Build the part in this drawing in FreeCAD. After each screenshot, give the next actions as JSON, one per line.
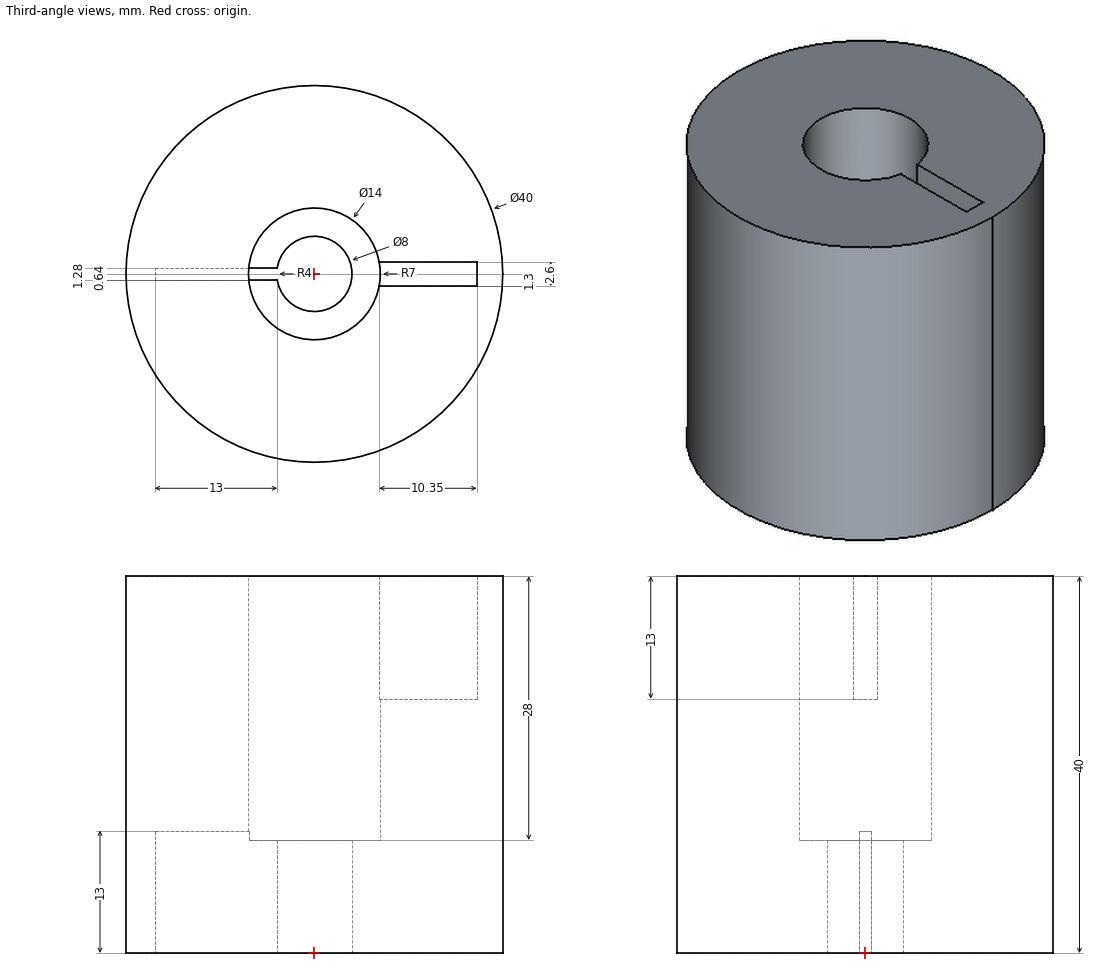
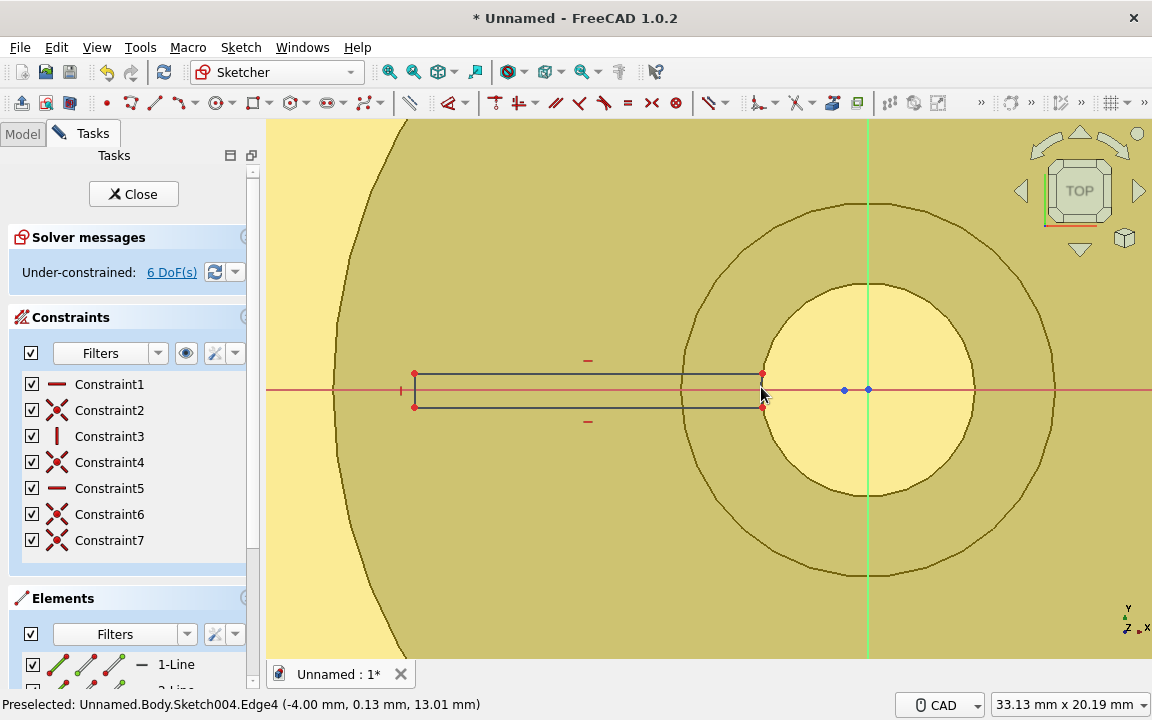
{"action": "left_click_drag", "start_coordinate": [835, 380], "coordinate": [878, 401]}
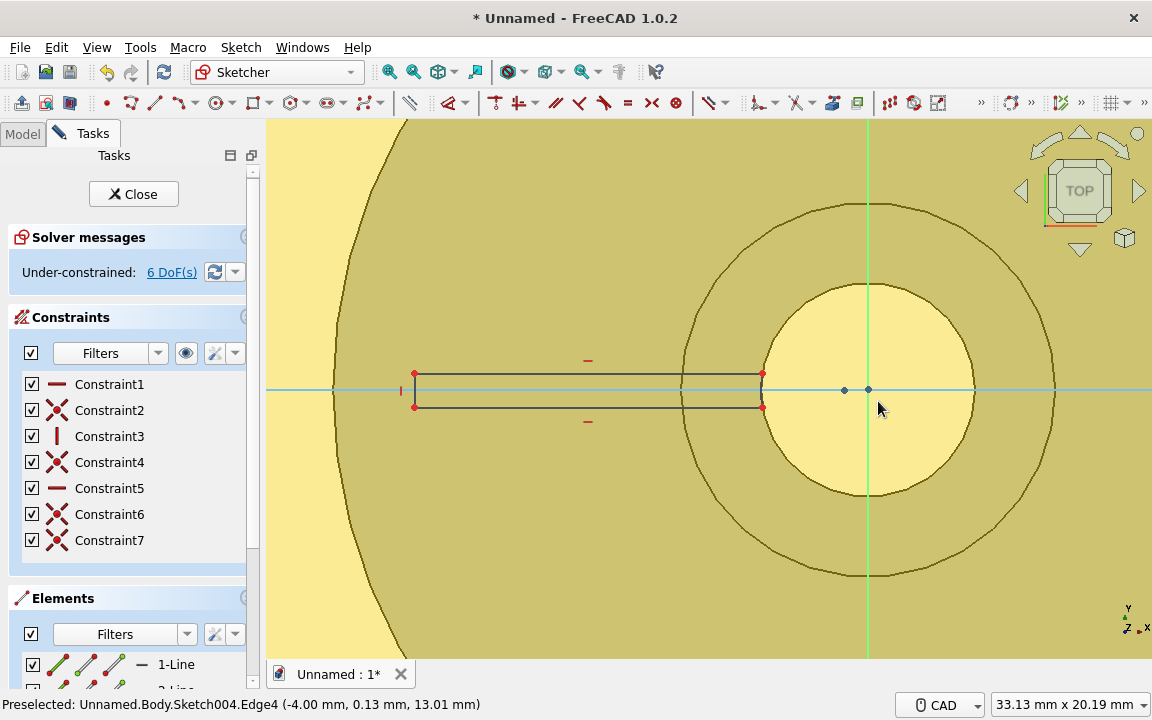
{"action": "key", "text": "c"}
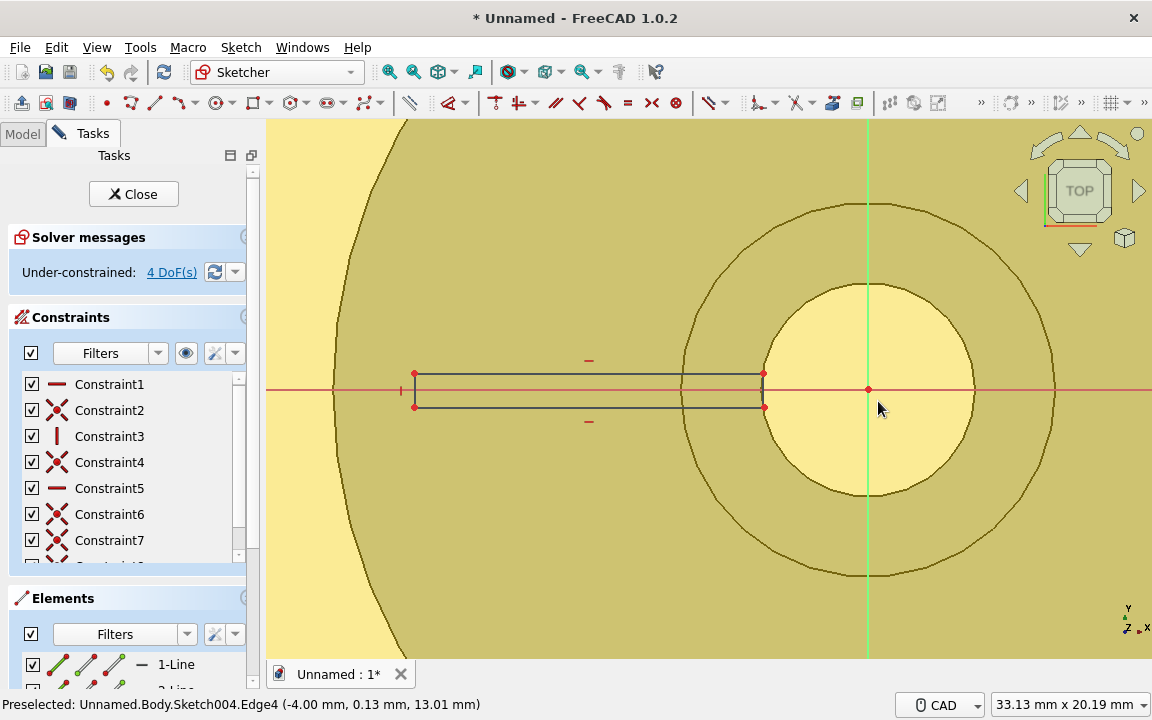
{"action": "key", "text": "d"}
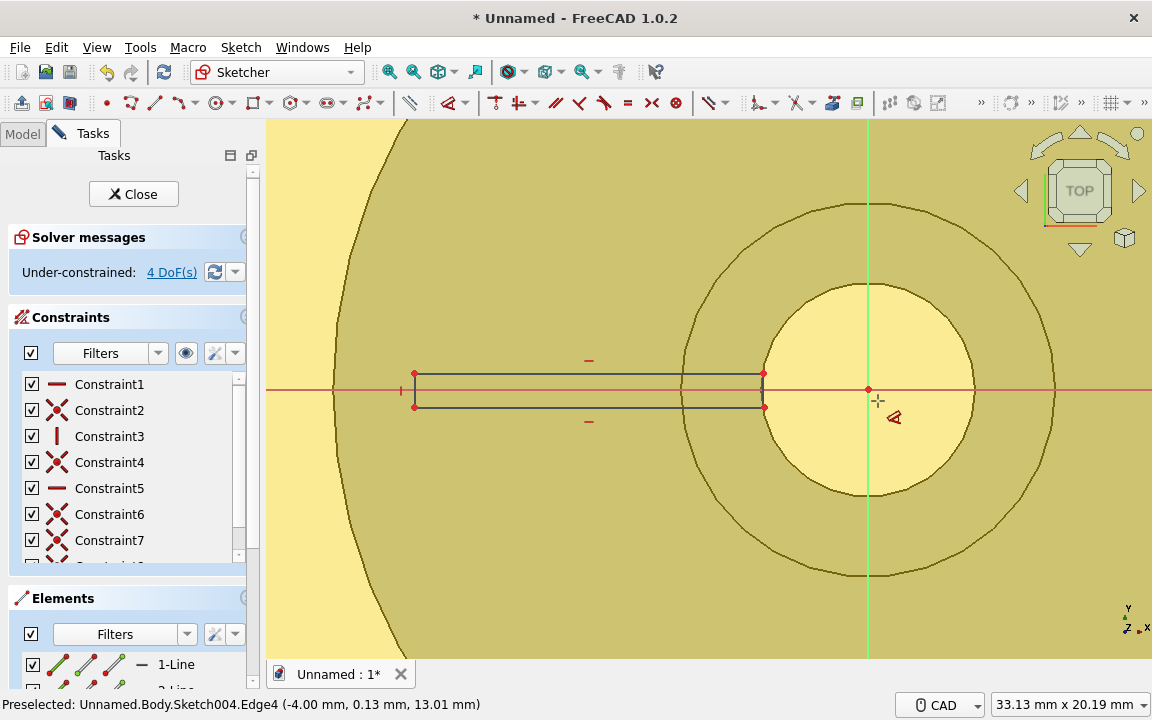
{"action": "left_click", "coordinate": [763, 391]}
{"action": "left_click", "coordinate": [747, 325]}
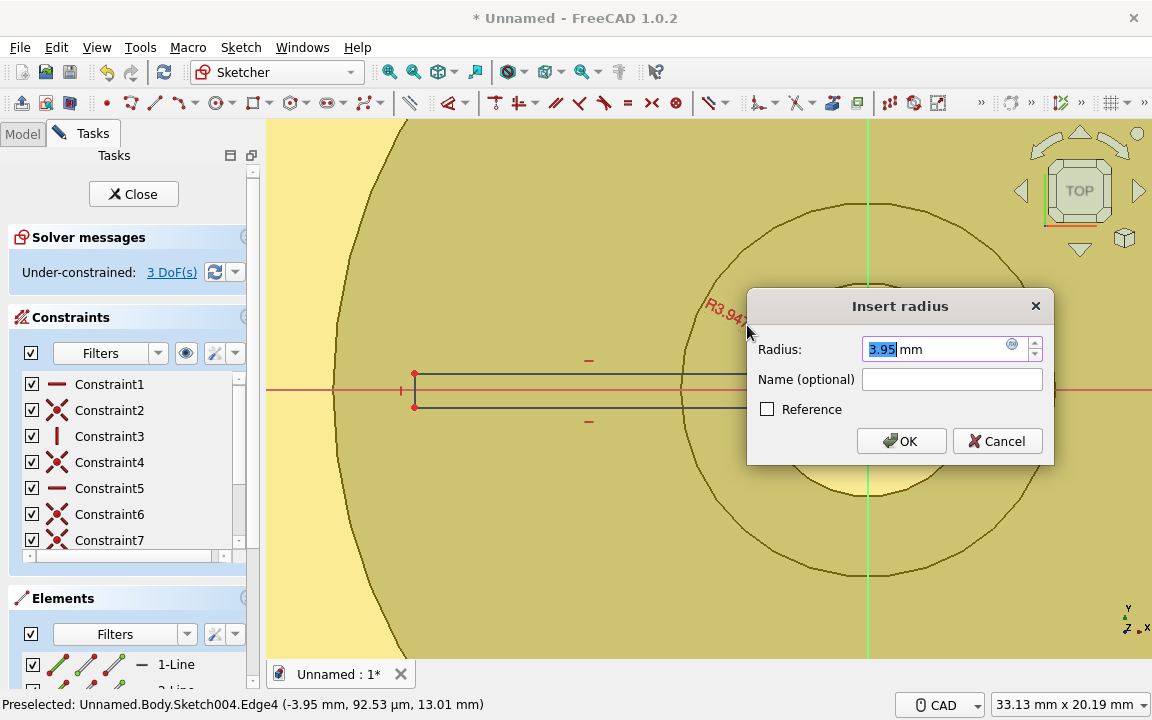
{"action": "type", "text": "4"}
{"action": "key", "text": "Return"}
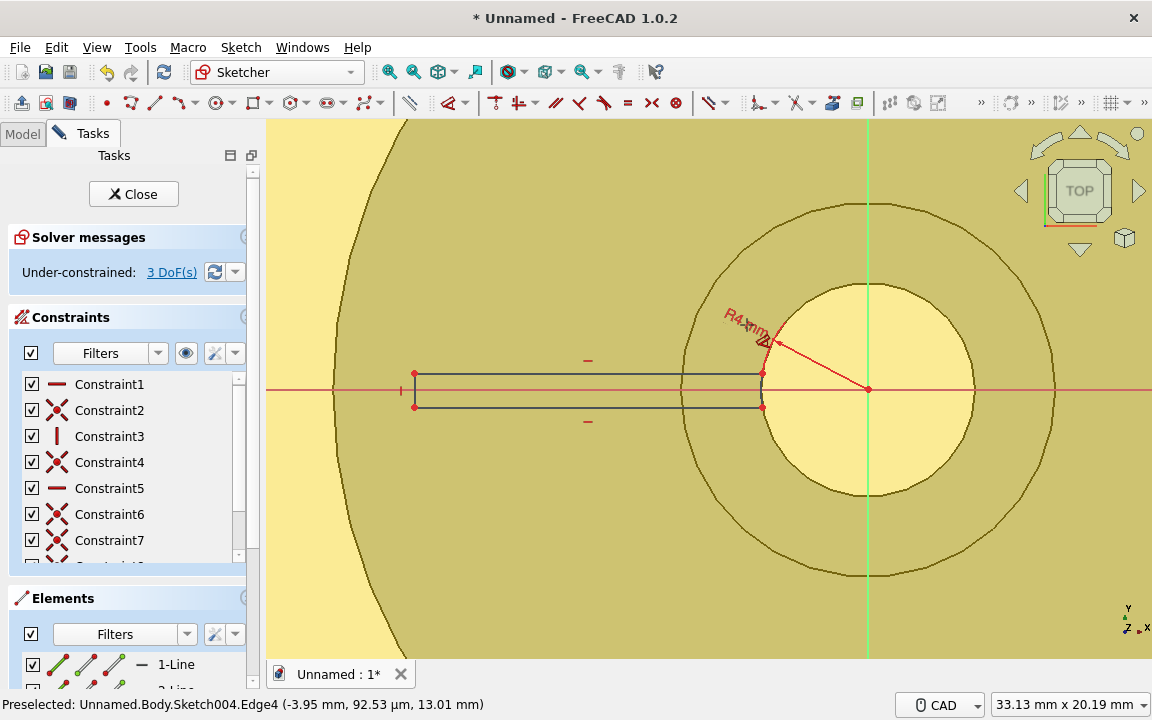
{"action": "left_click", "coordinate": [658, 408]}
{"action": "left_click", "coordinate": [589, 442]}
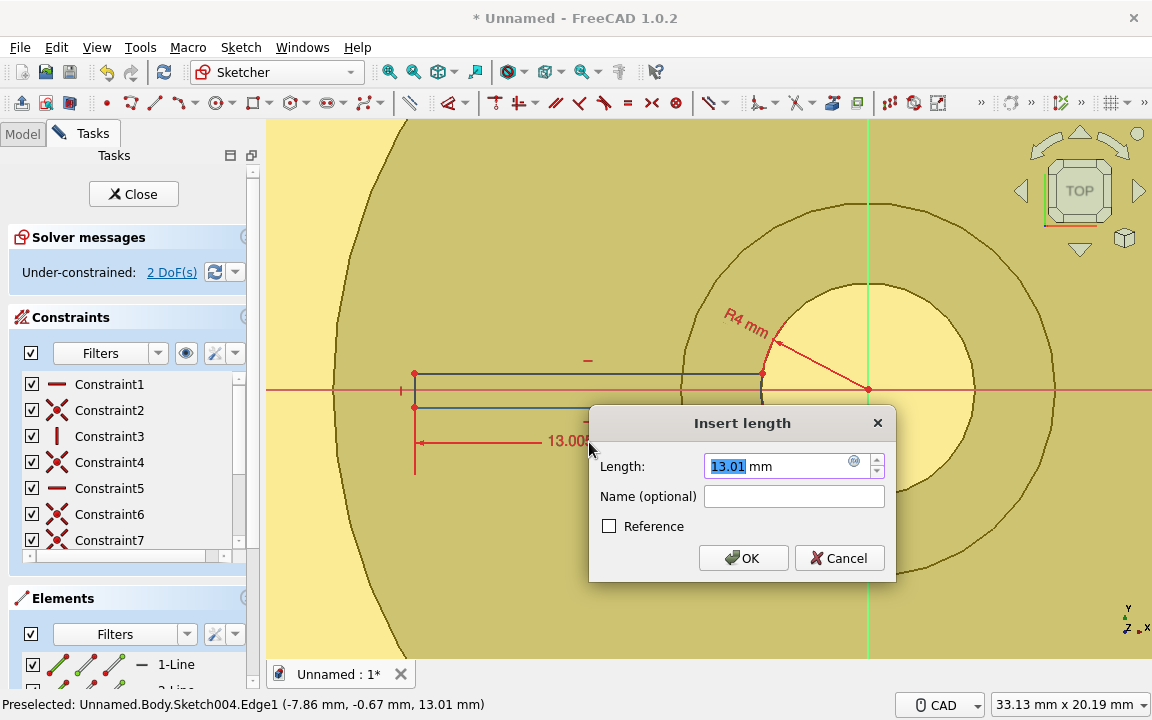
{"action": "type", "text": "13"}
{"action": "key", "text": "Return"}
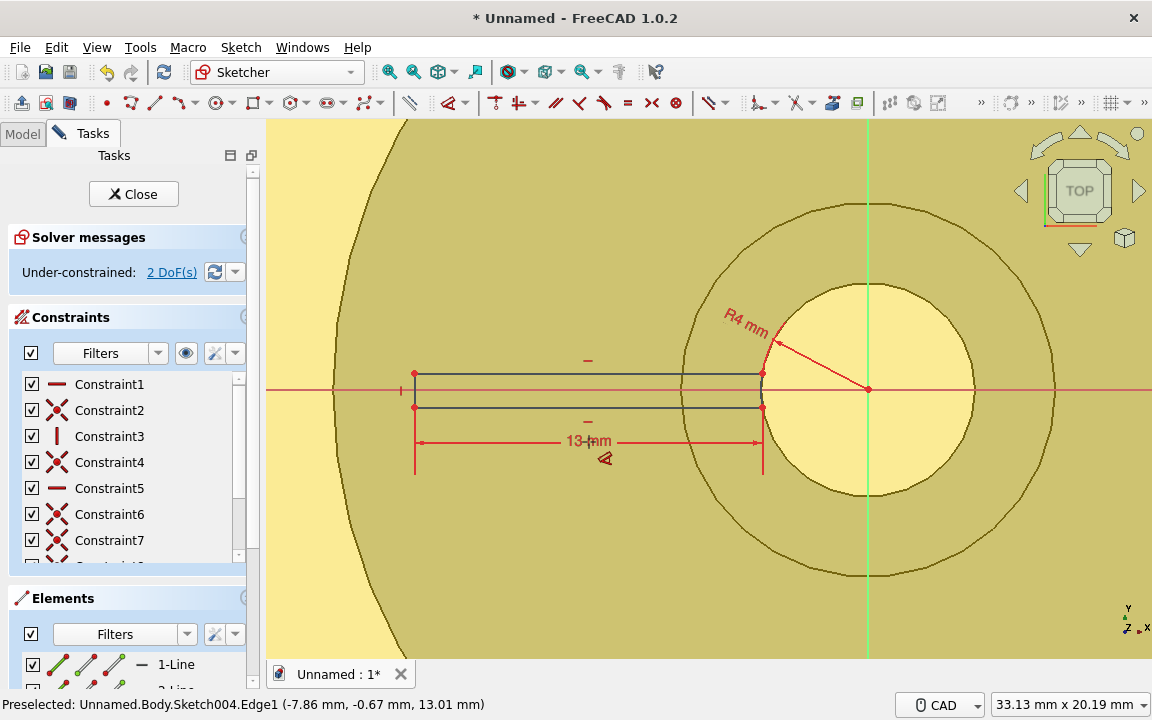
{"action": "left_click", "coordinate": [415, 387]}
{"action": "left_click", "coordinate": [381, 383]}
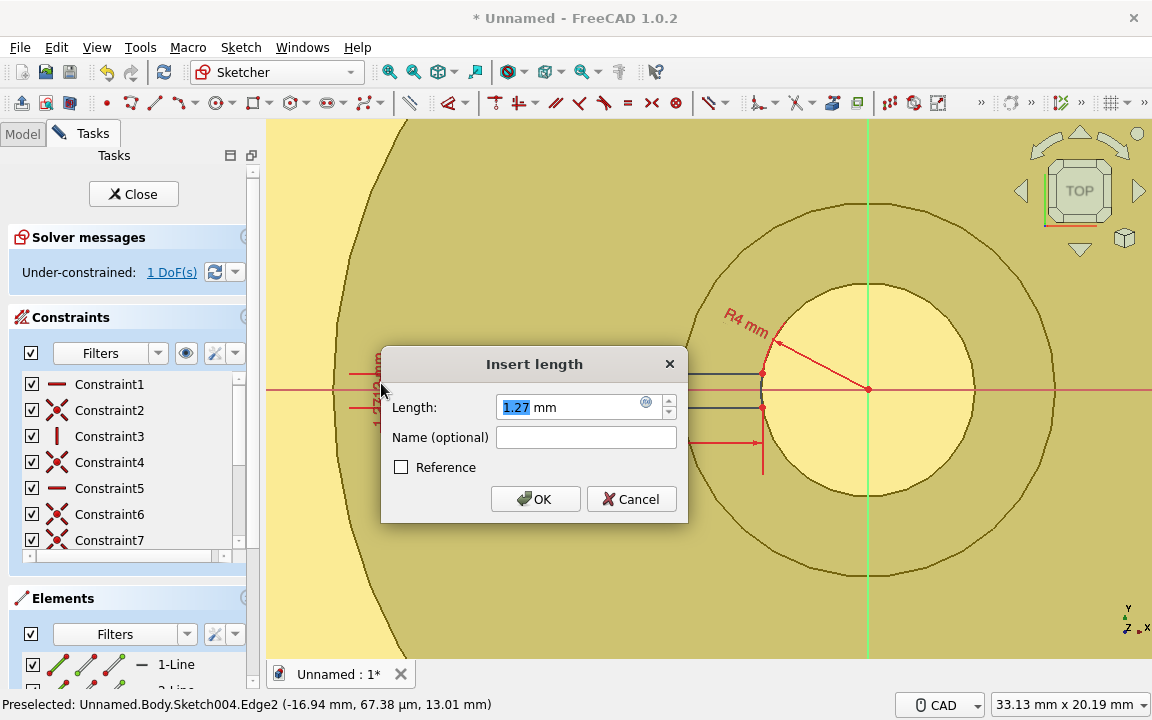
{"action": "type", "text": "1.28"}
{"action": "key", "text": "Return"}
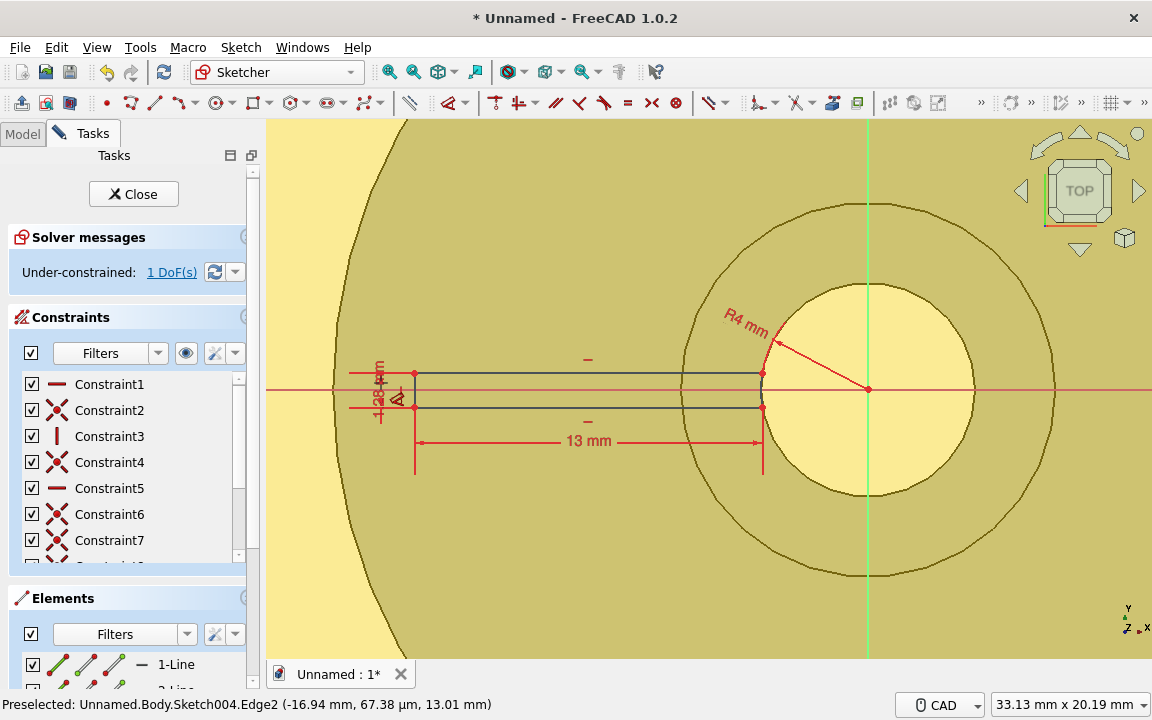
{"action": "scroll", "coordinate": [763, 408], "scroll_direction": "up", "scroll_amount": 5}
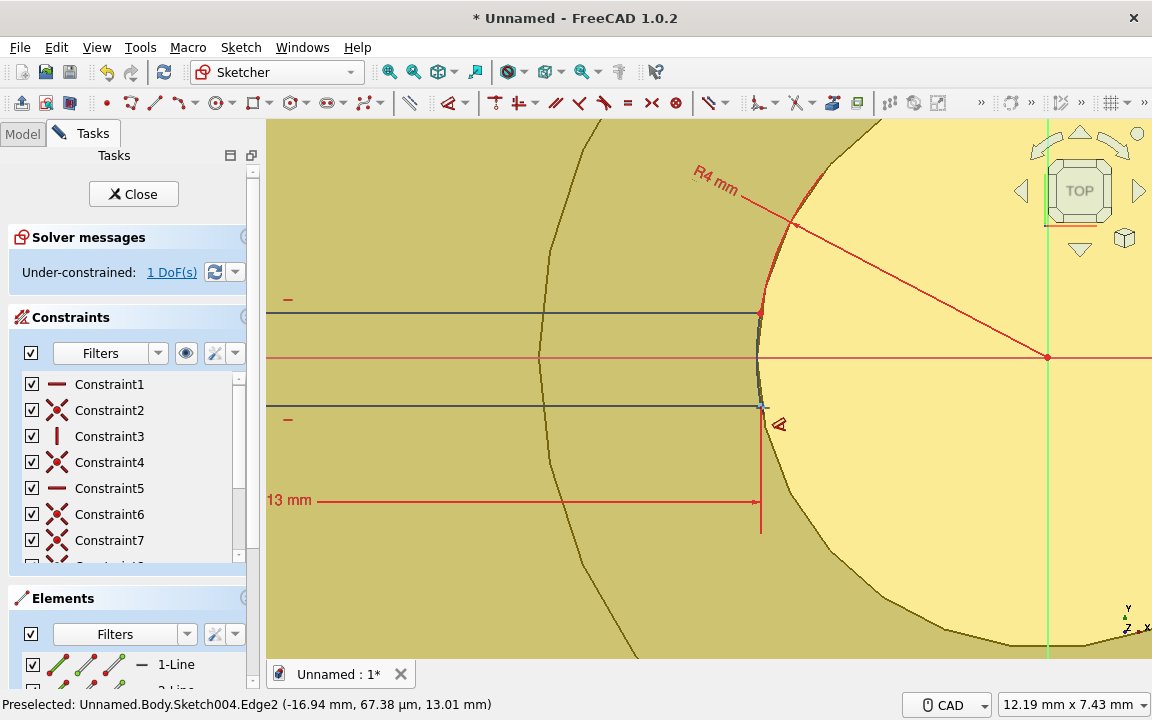
{"action": "left_click", "coordinate": [761, 406]}
{"action": "left_click", "coordinate": [727, 382]}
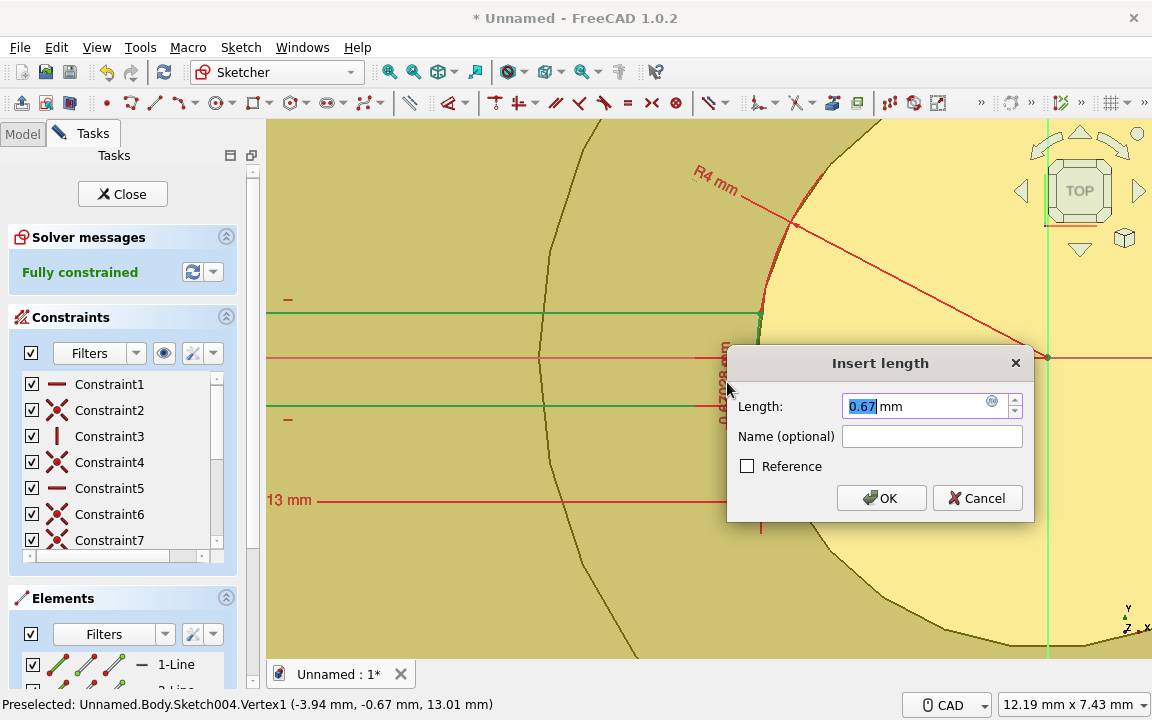
{"action": "type", "text": "0.64"}
{"action": "key", "text": "Return"}
{"action": "key", "text": "Escape"}